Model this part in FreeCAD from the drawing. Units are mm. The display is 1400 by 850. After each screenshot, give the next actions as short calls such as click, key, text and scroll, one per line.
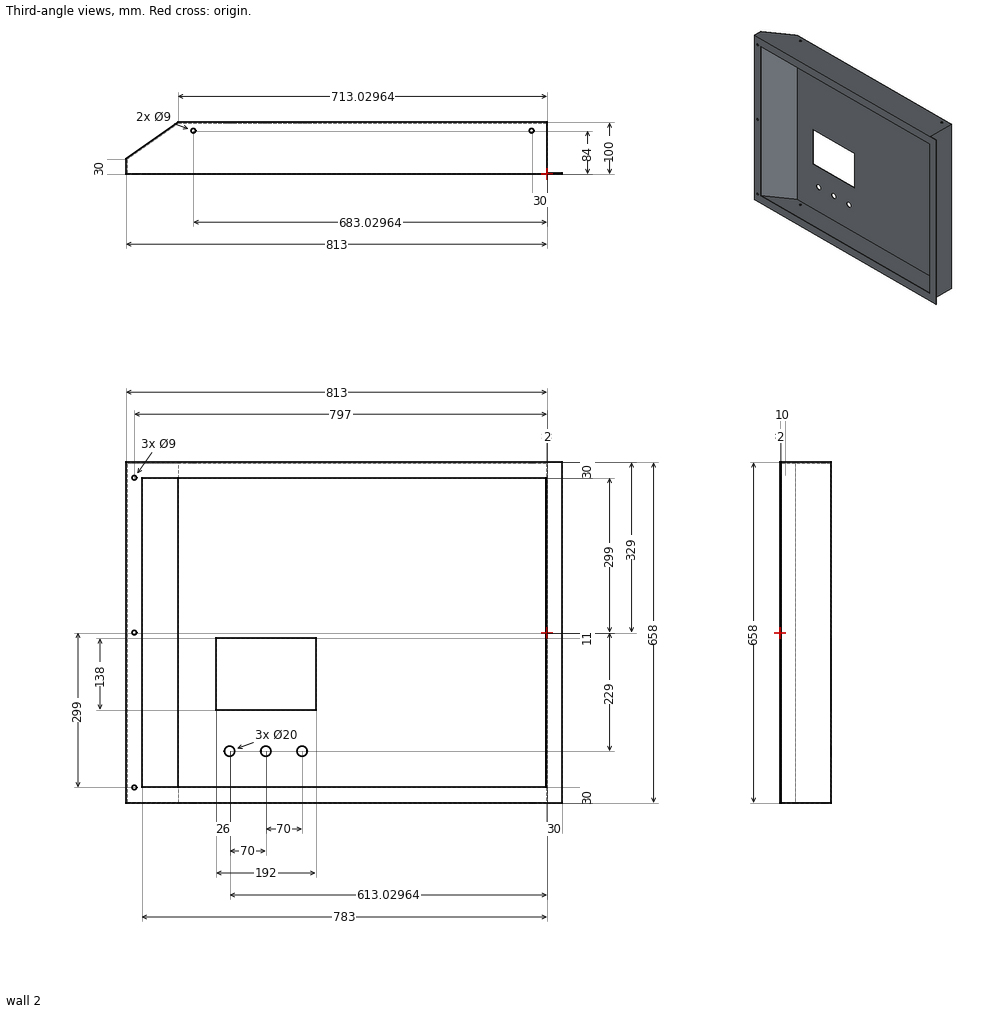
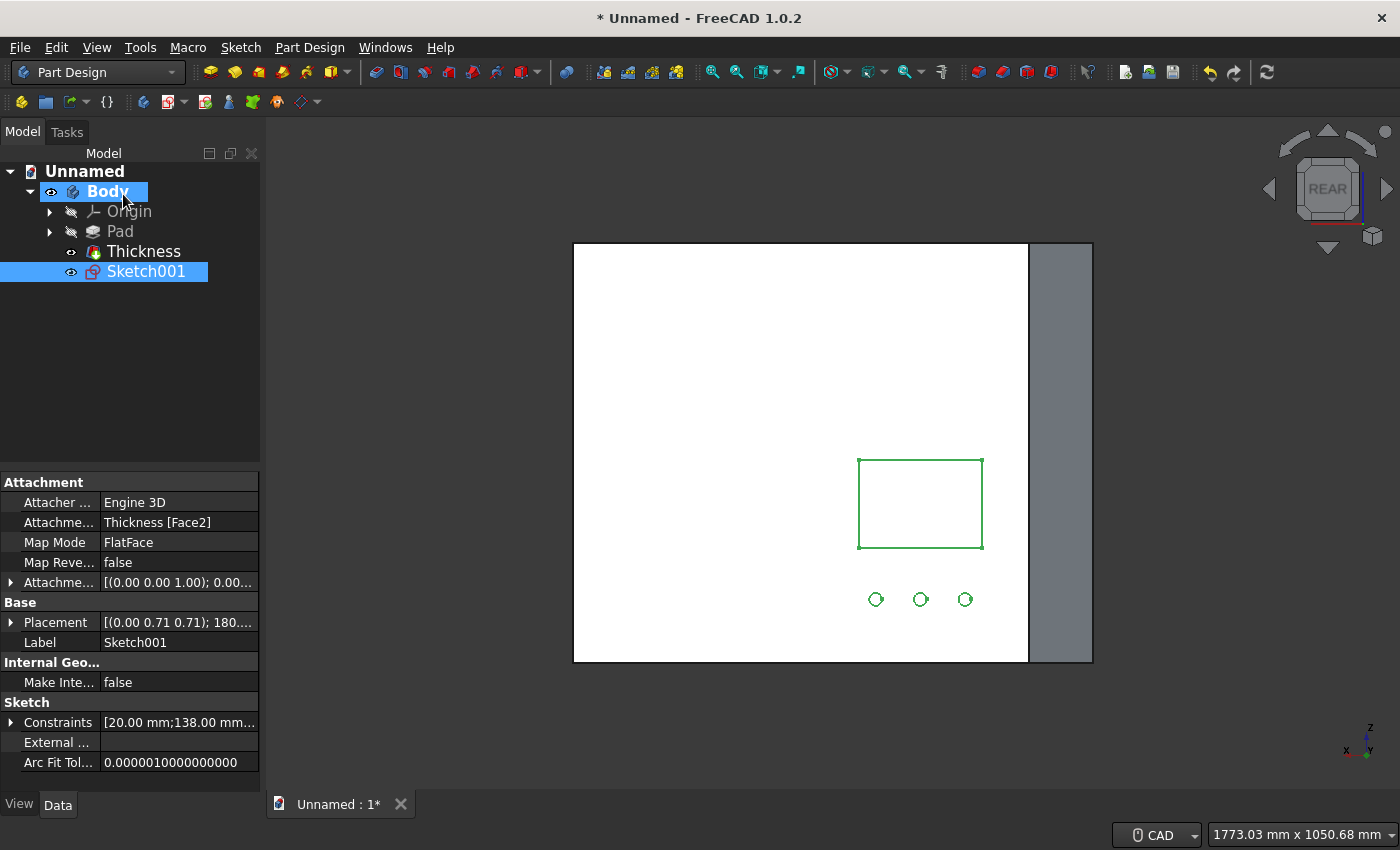
click(378, 72)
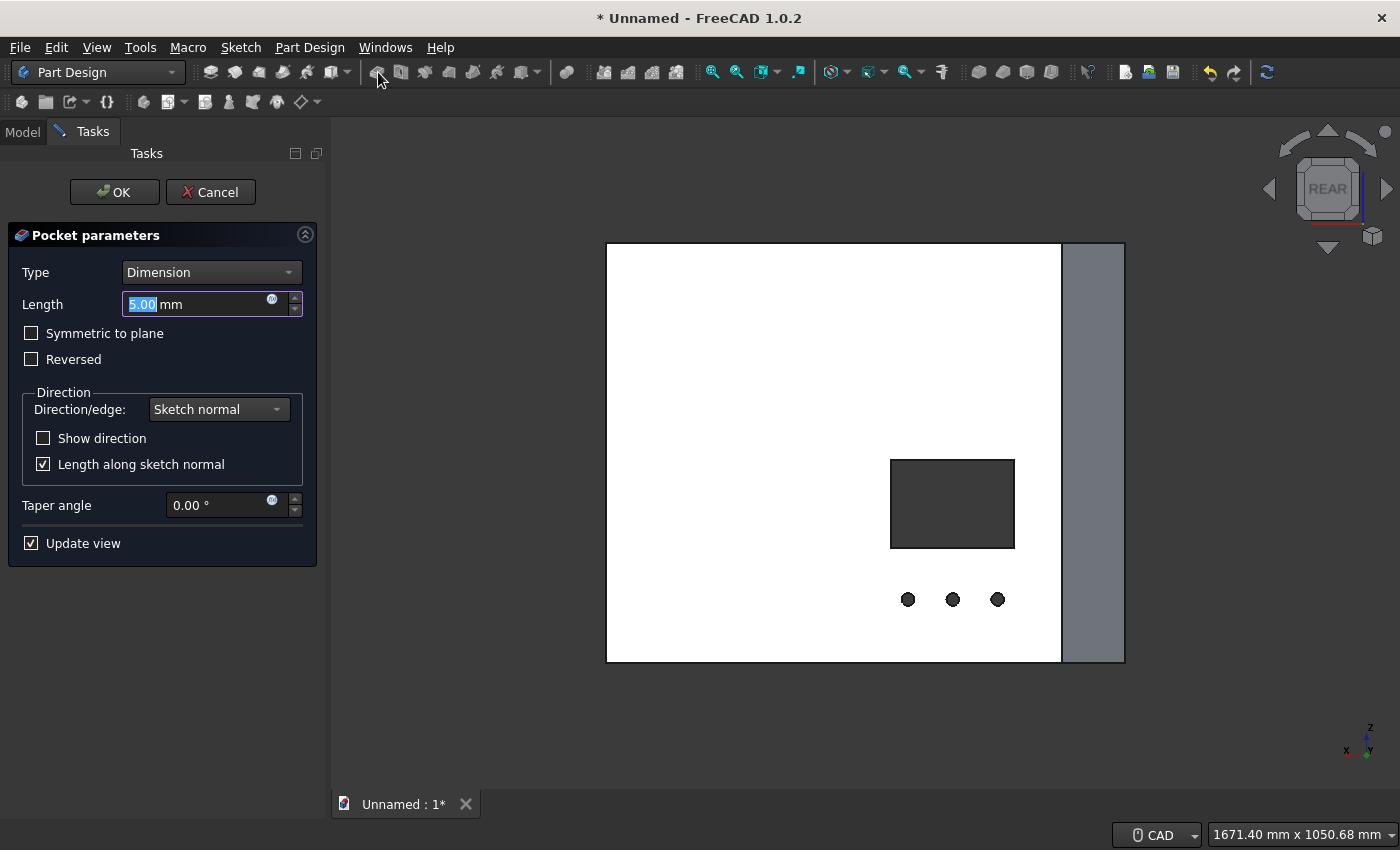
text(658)
key(Tab)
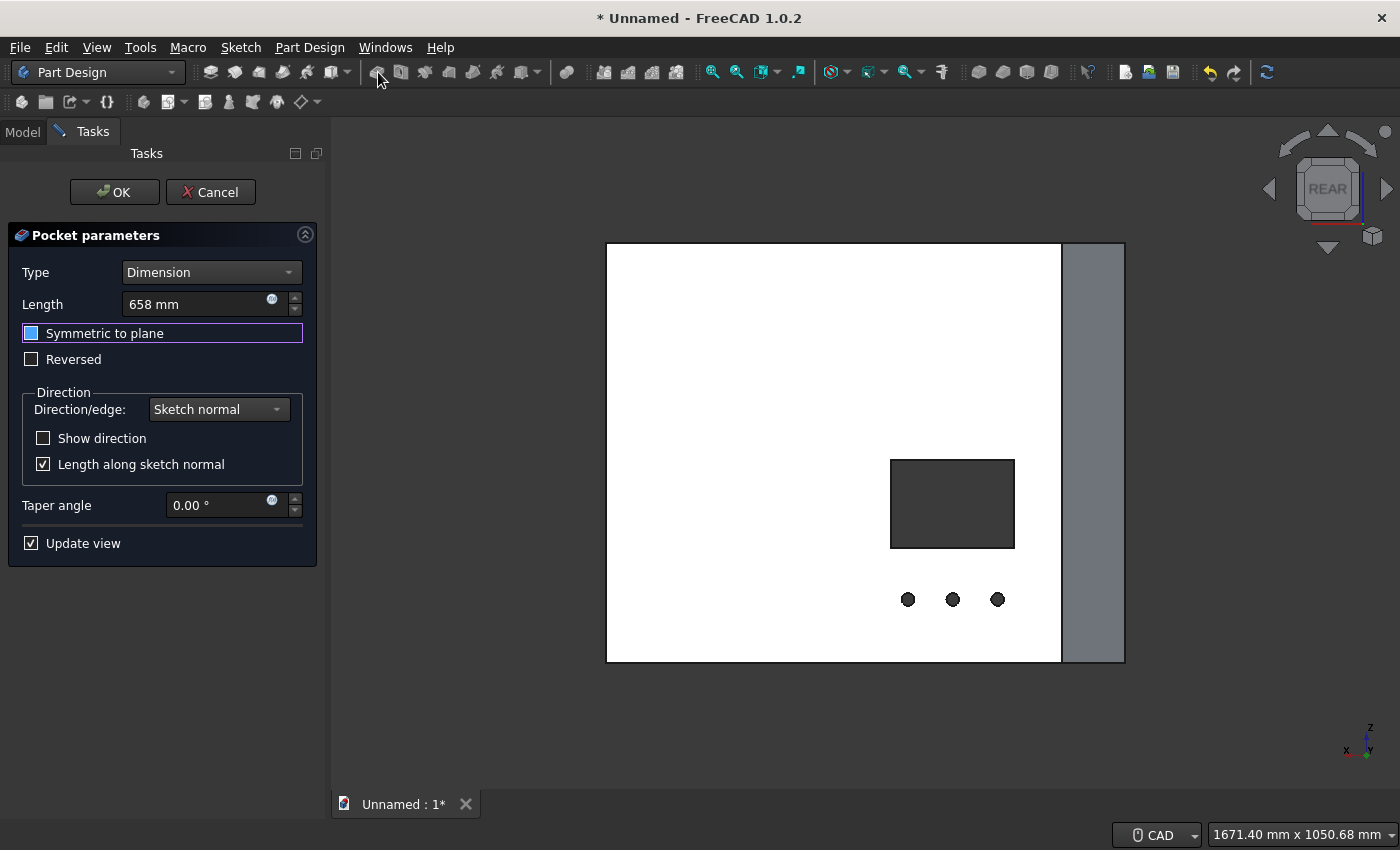
click(115, 192)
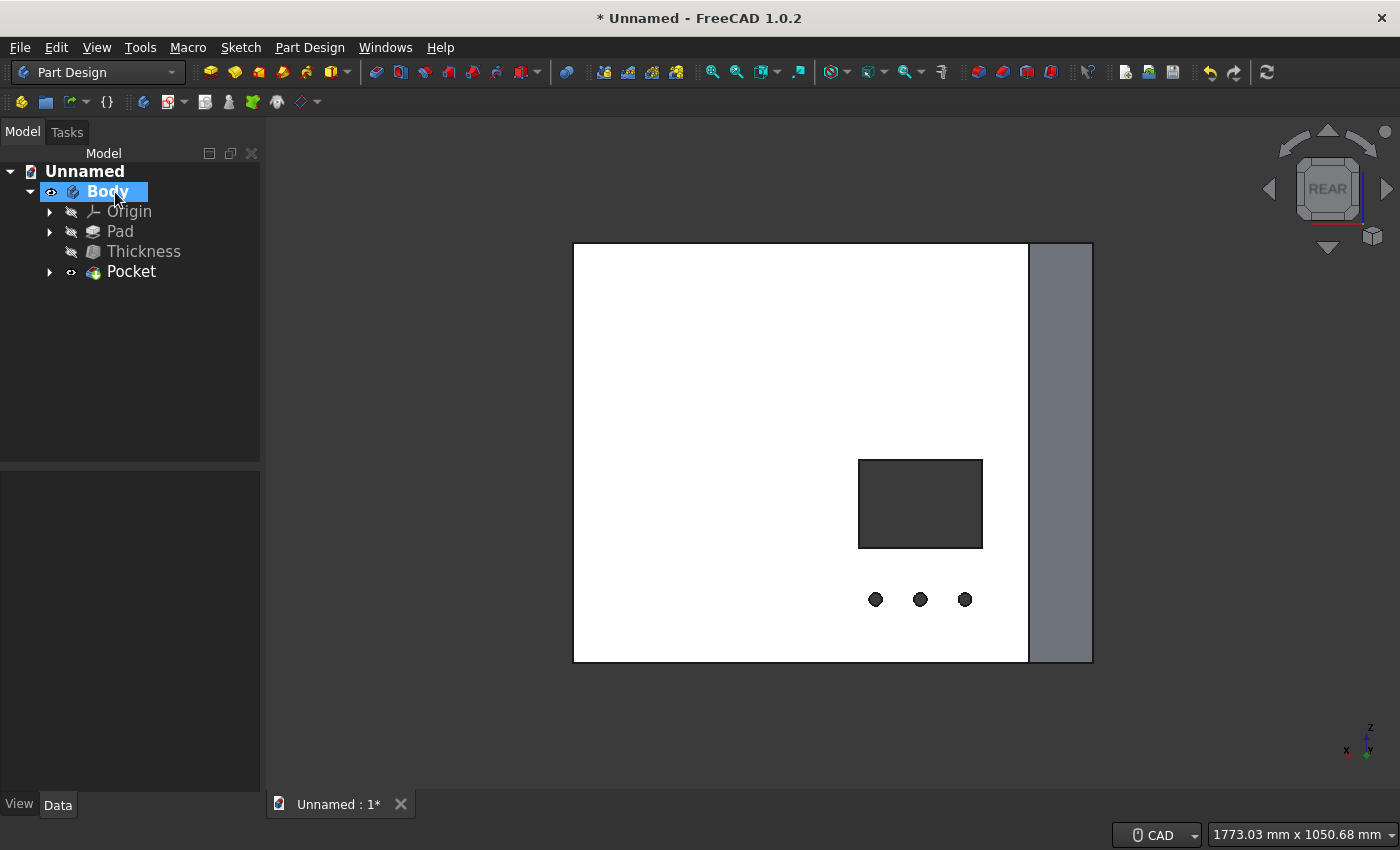
click(168, 102)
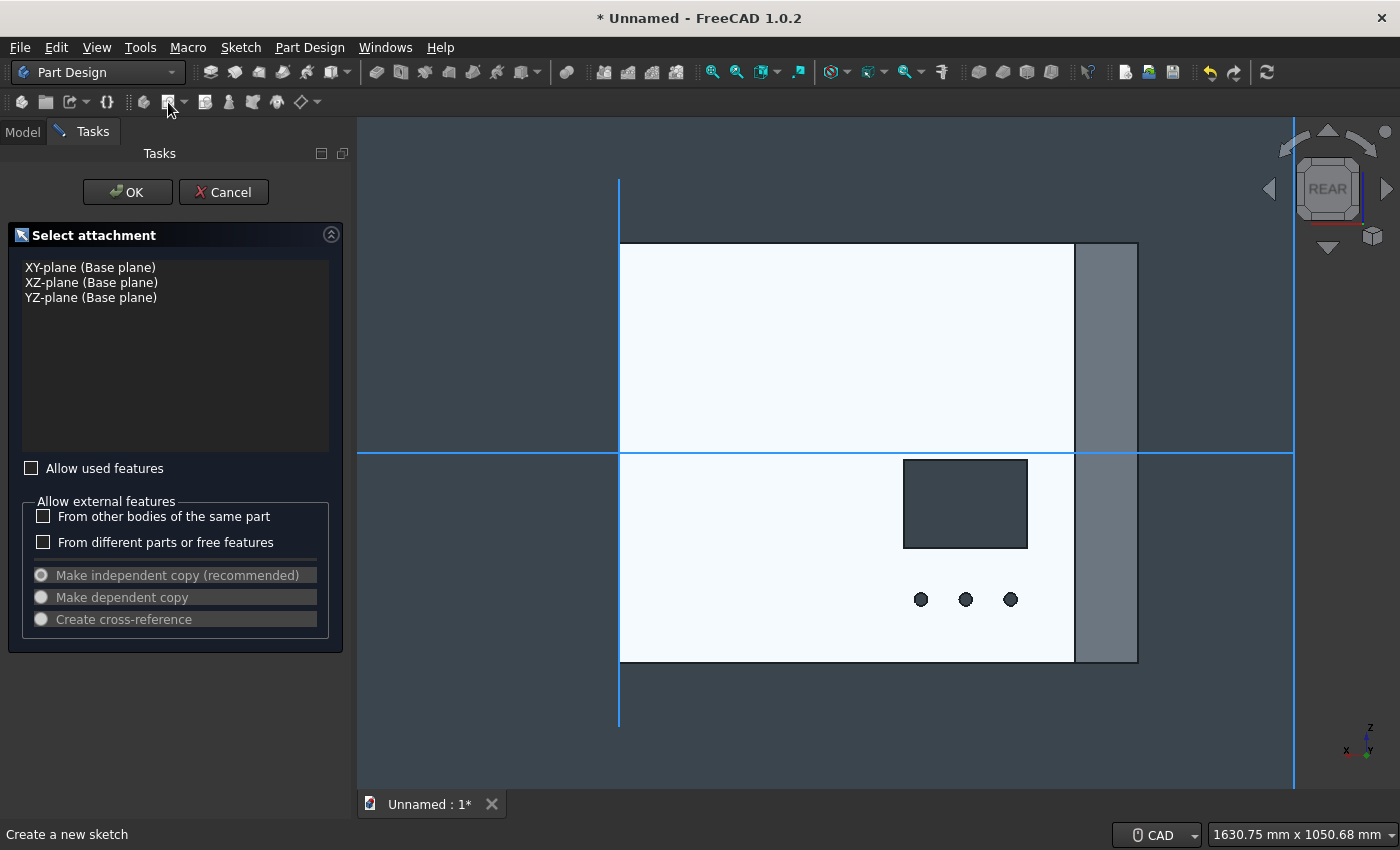
click(82, 282)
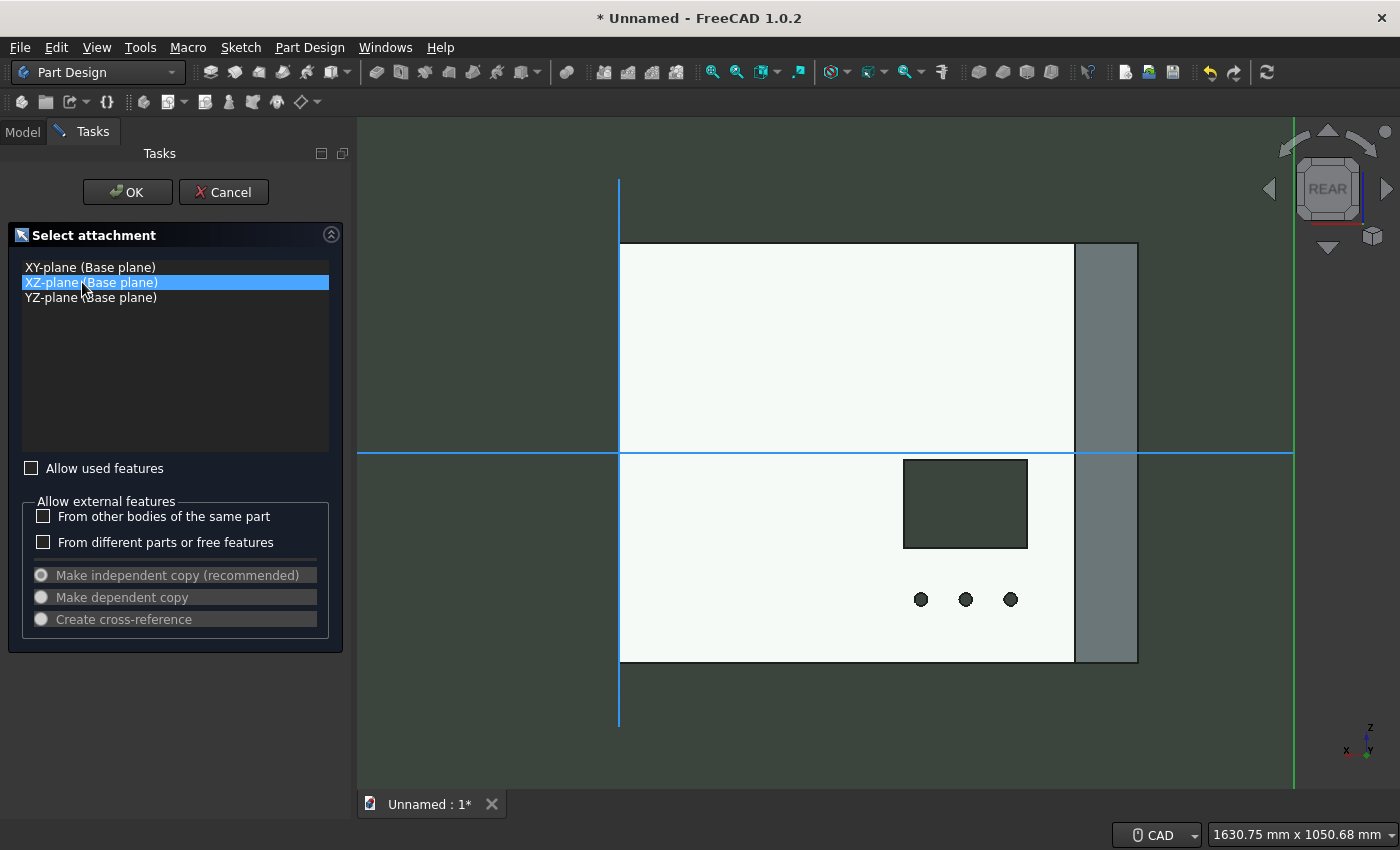
click(128, 192)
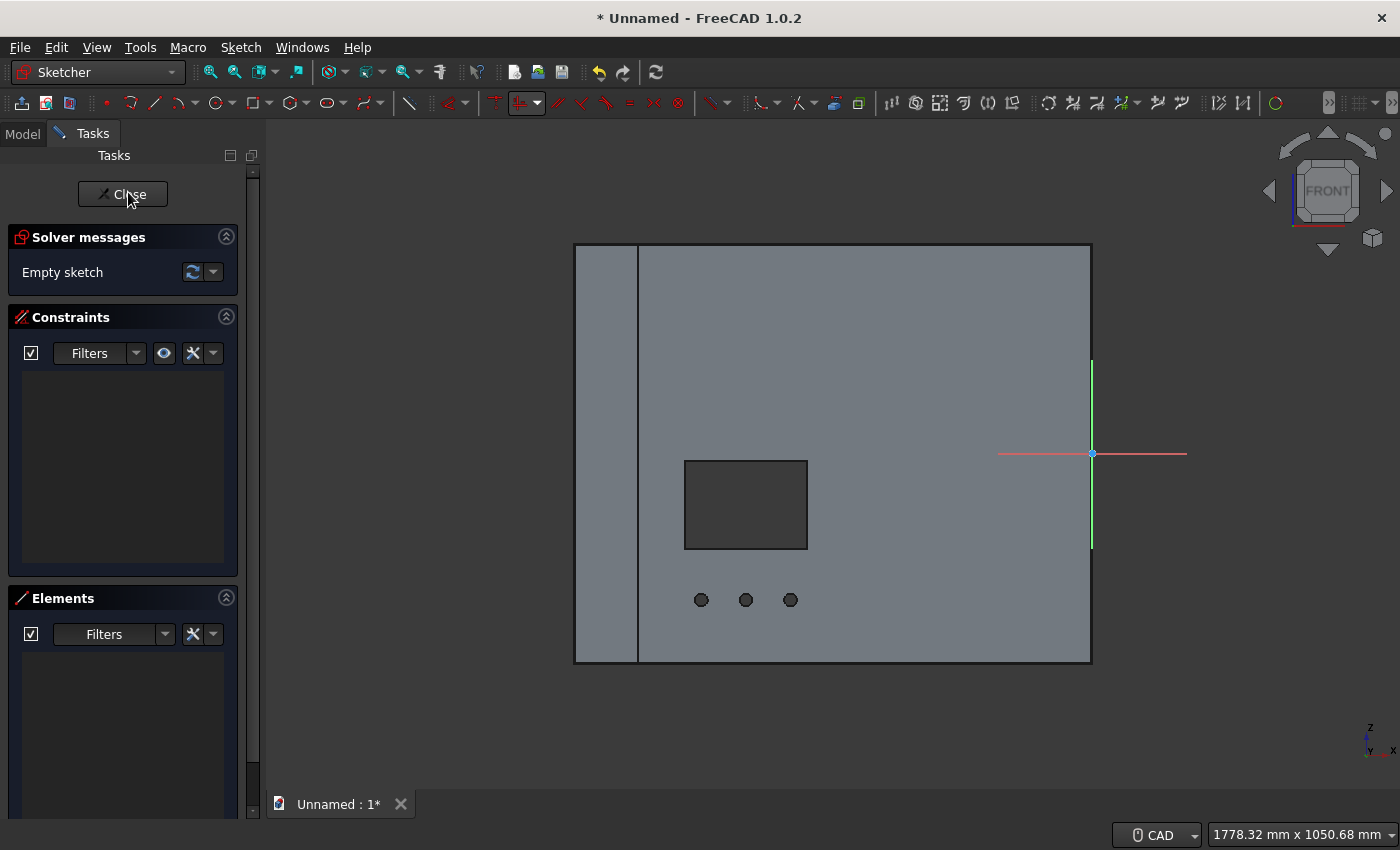
click(254, 104)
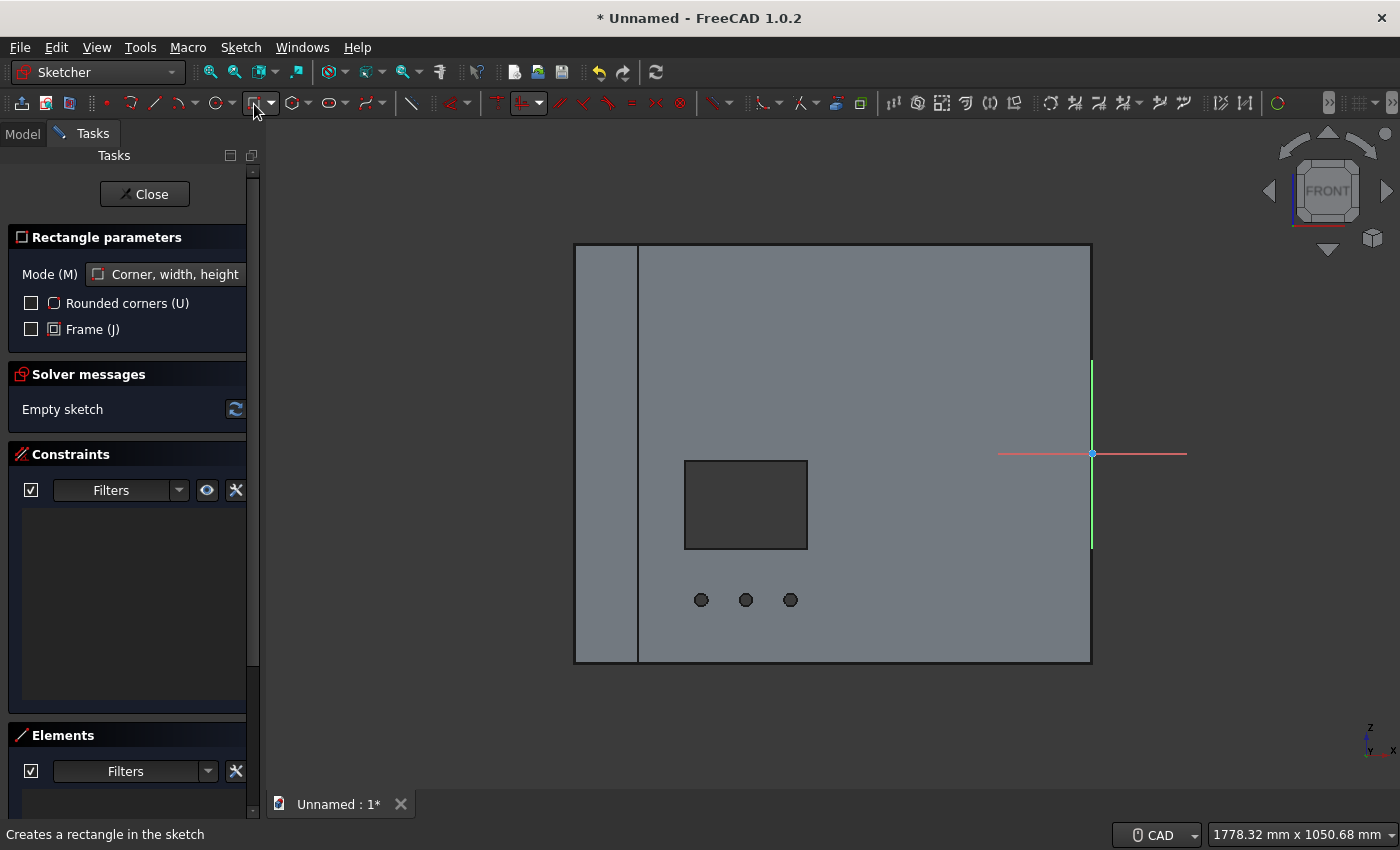
scroll(1091, 244, up, 13)